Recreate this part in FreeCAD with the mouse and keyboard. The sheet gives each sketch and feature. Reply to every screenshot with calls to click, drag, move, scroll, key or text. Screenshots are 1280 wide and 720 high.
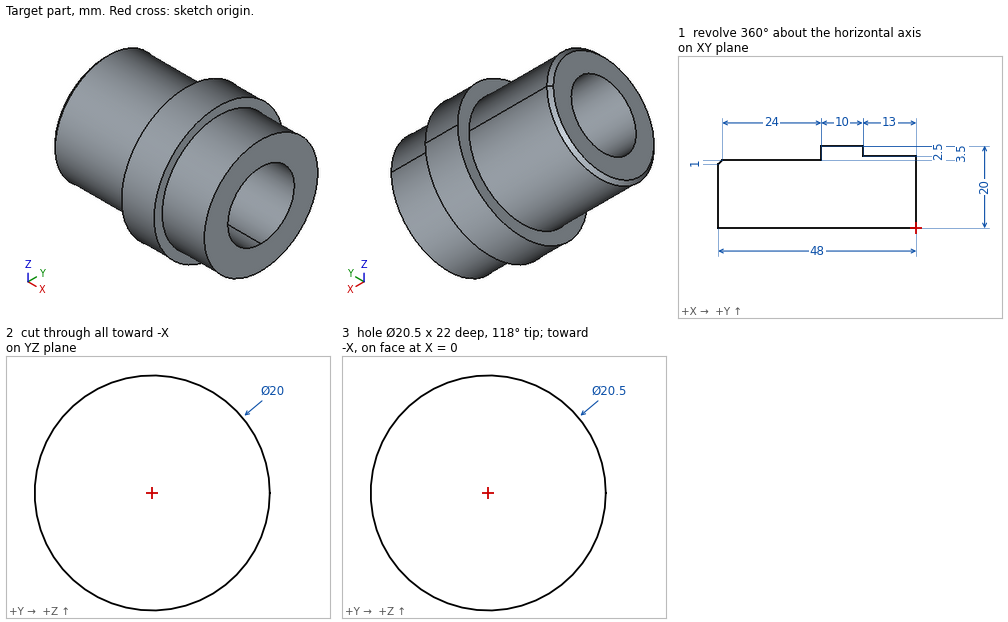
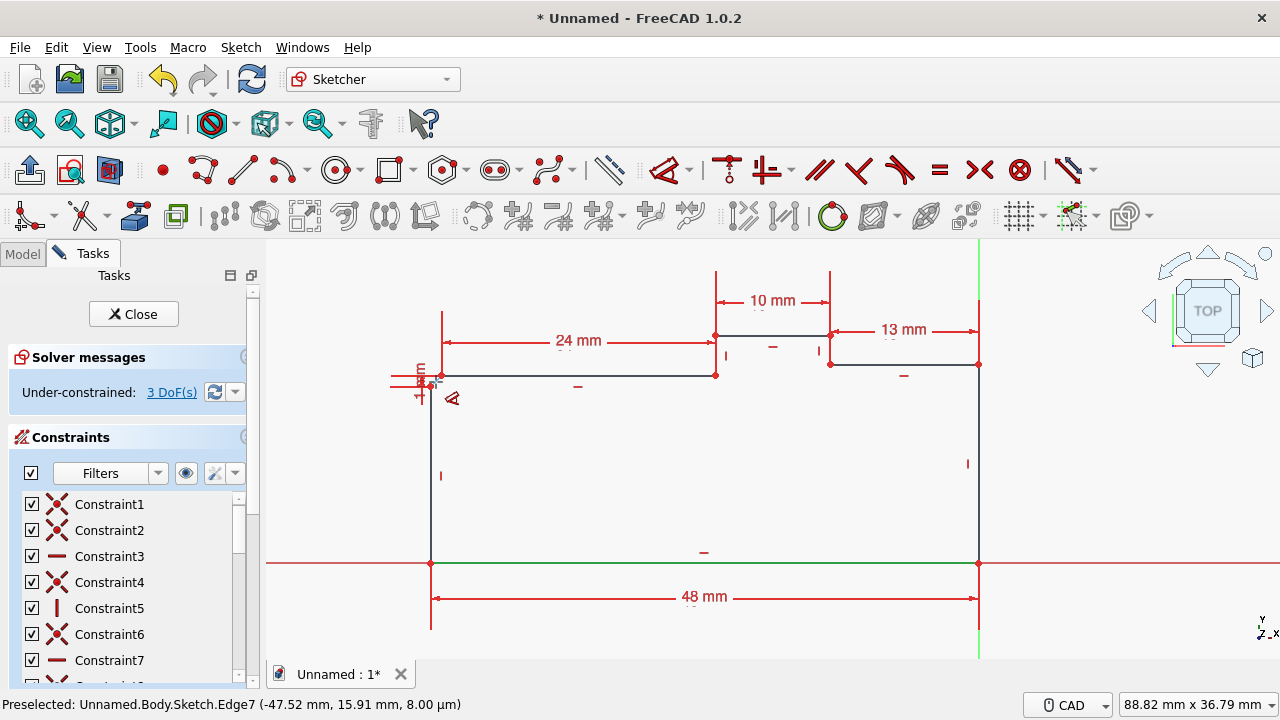
scroll(830, 356, up, 3)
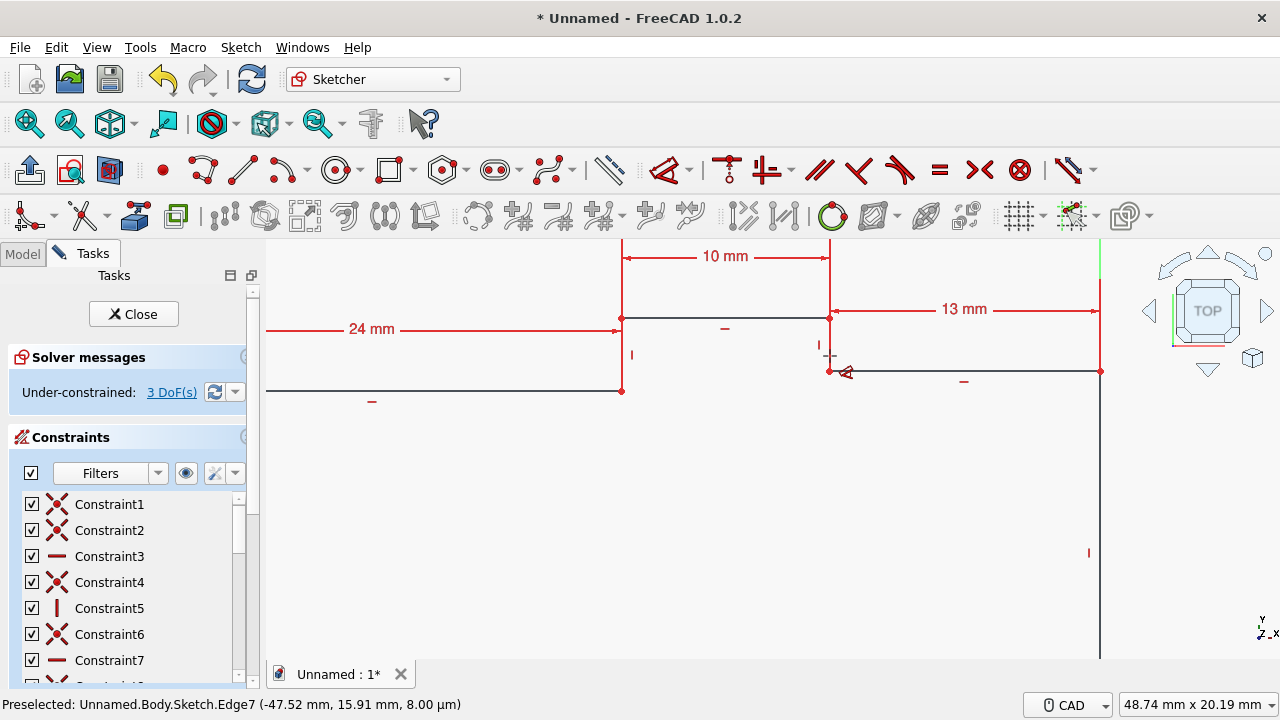
click(830, 355)
click(864, 345)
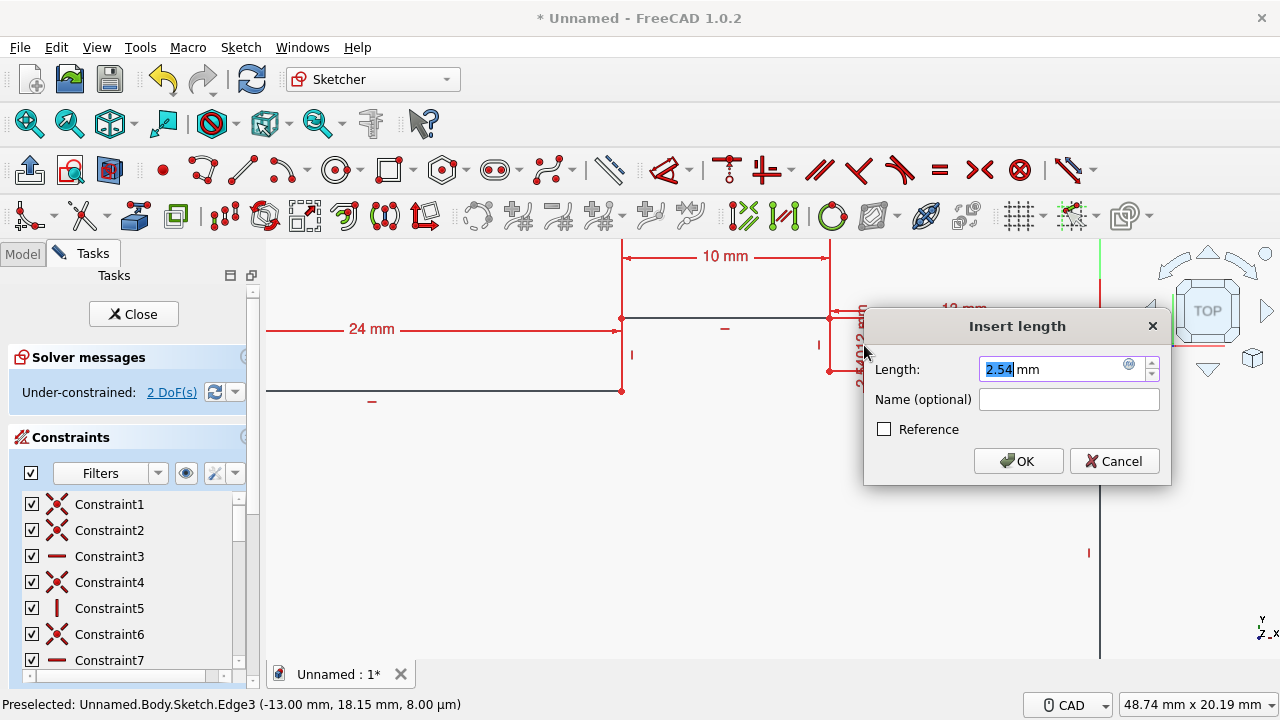
text(2.5)
key(Return)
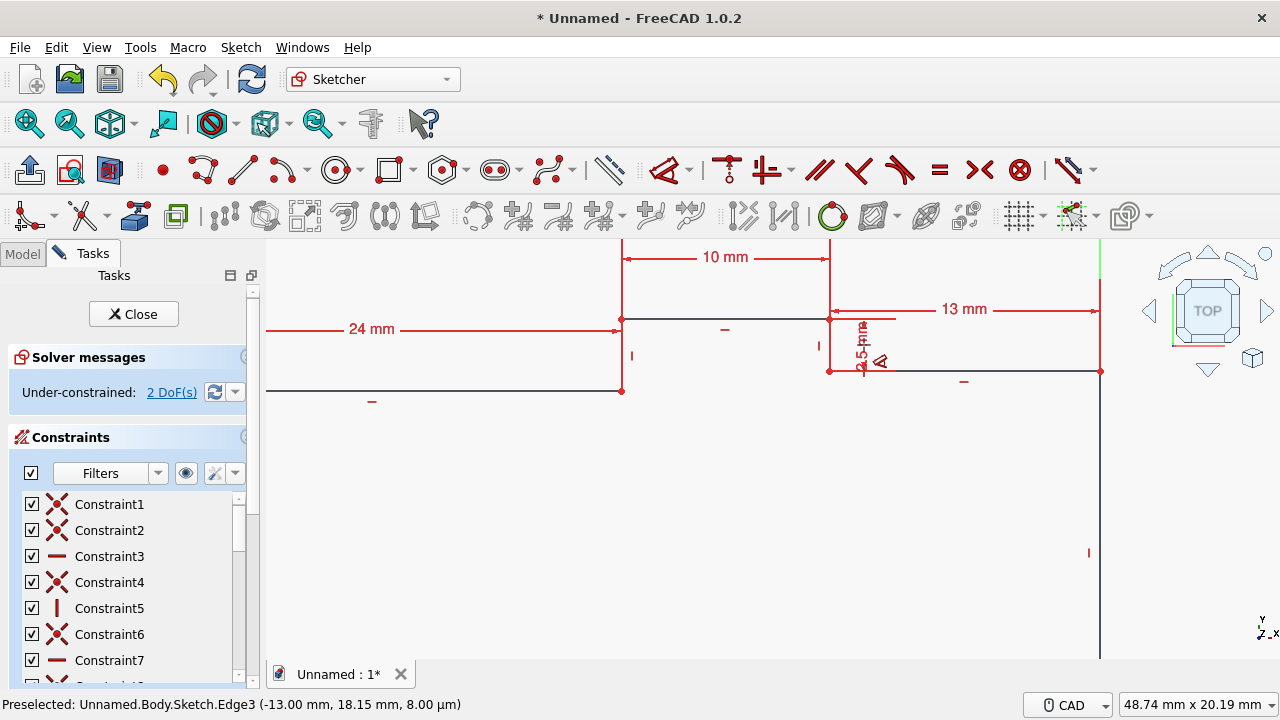
click(622, 341)
click(656, 355)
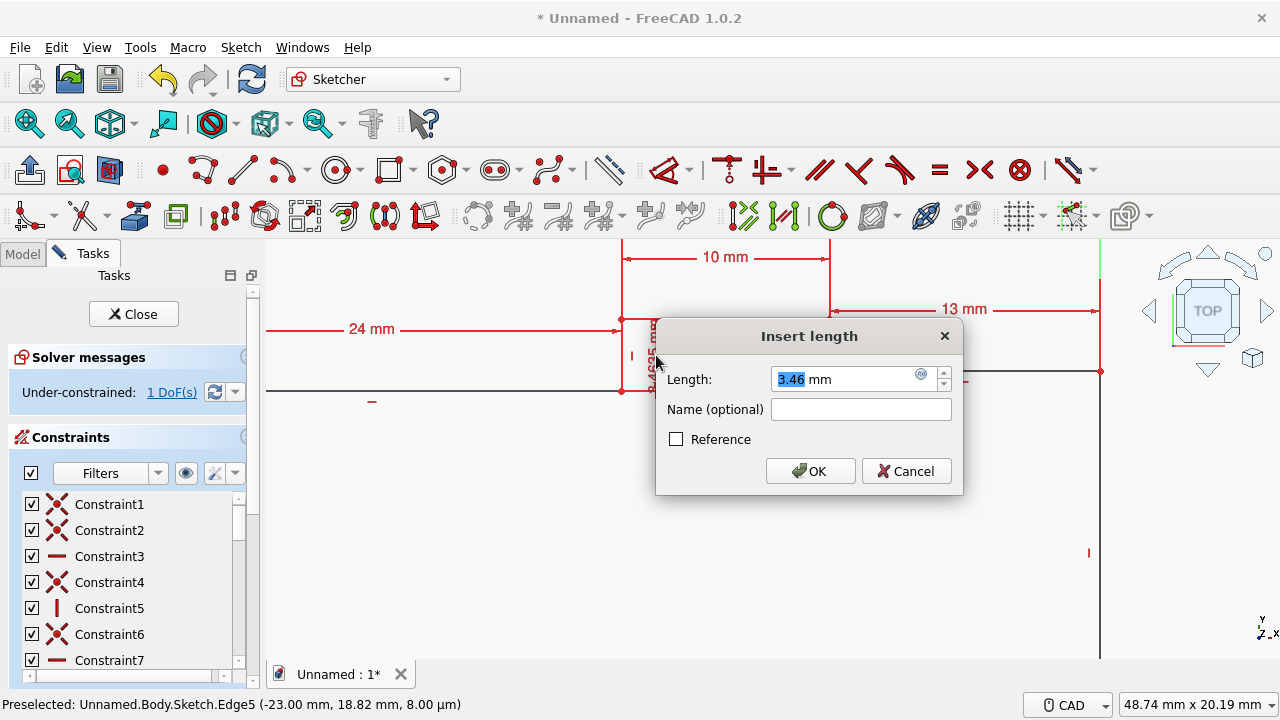
text(3.5)
key(Return)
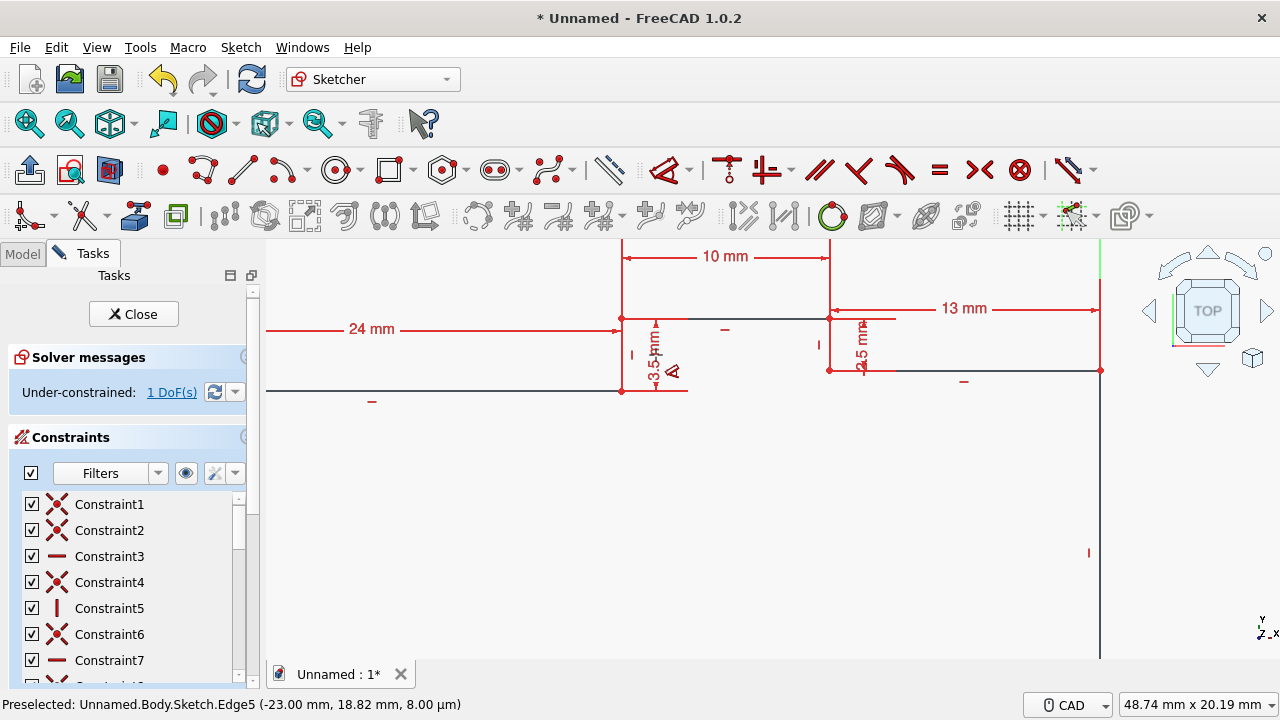
click(830, 319)
click(796, 475)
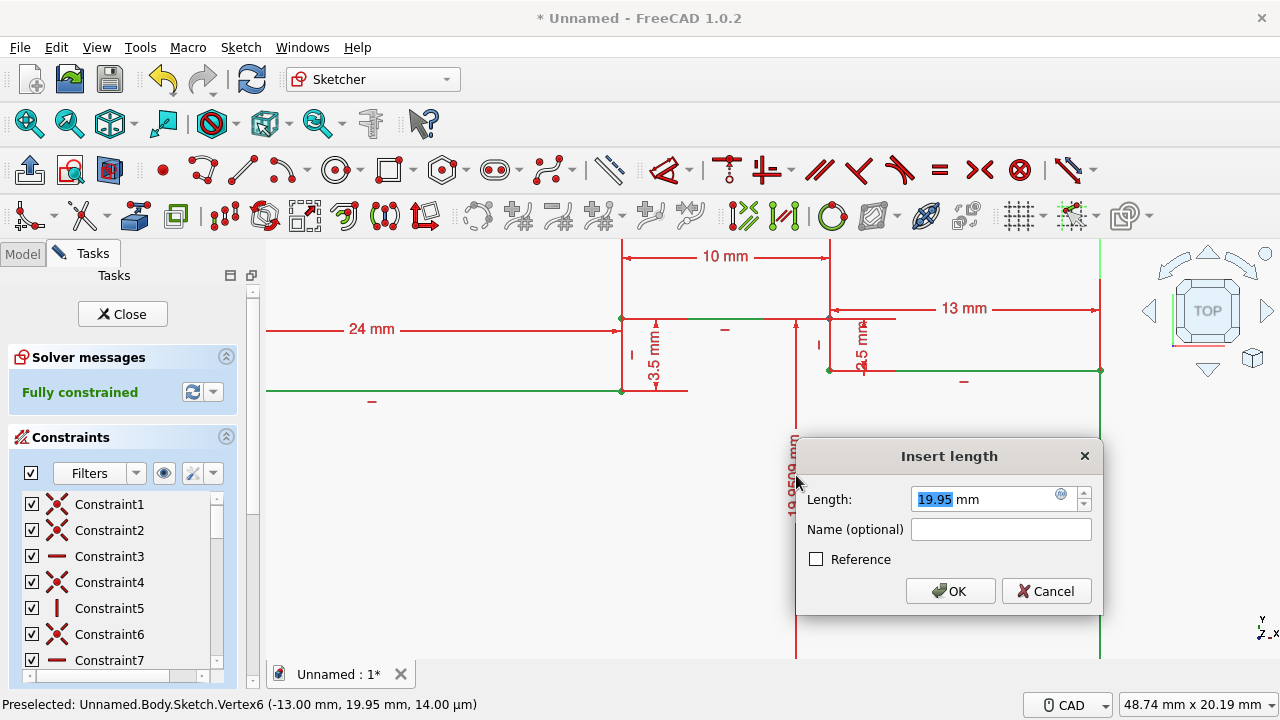
text(20)
key(Return)
key(Escape)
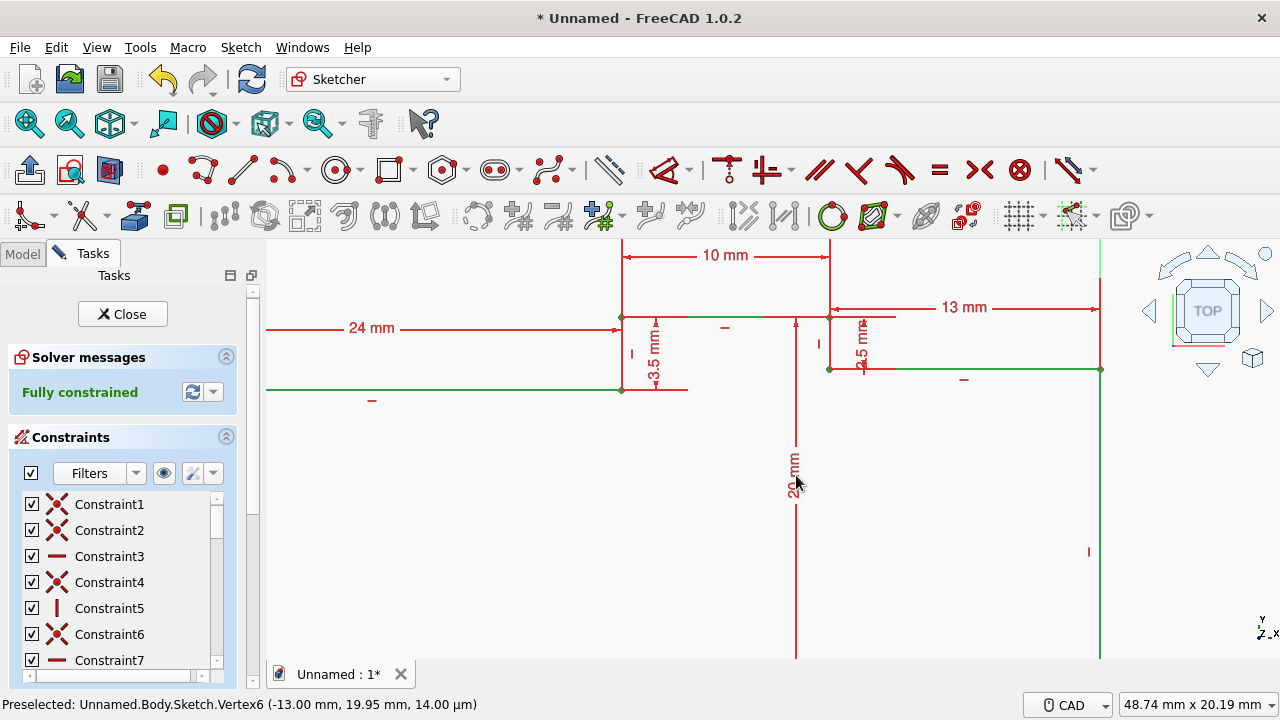
click(123, 314)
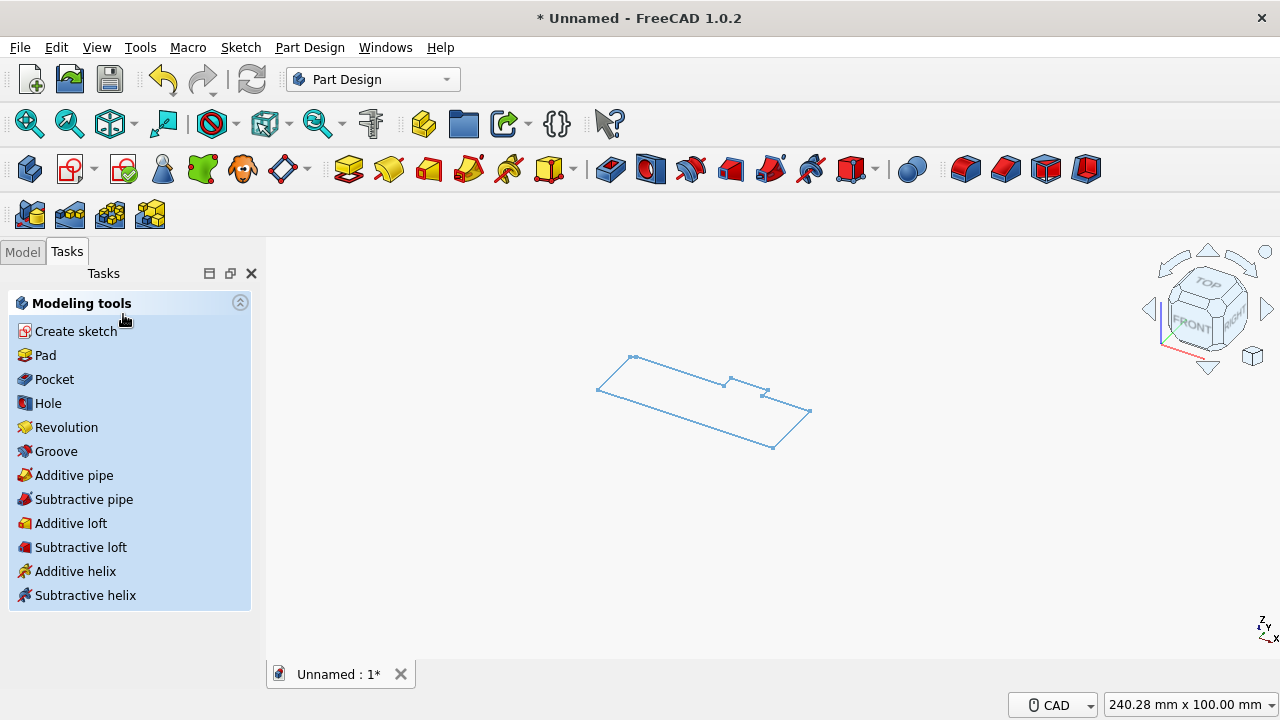
click(390, 170)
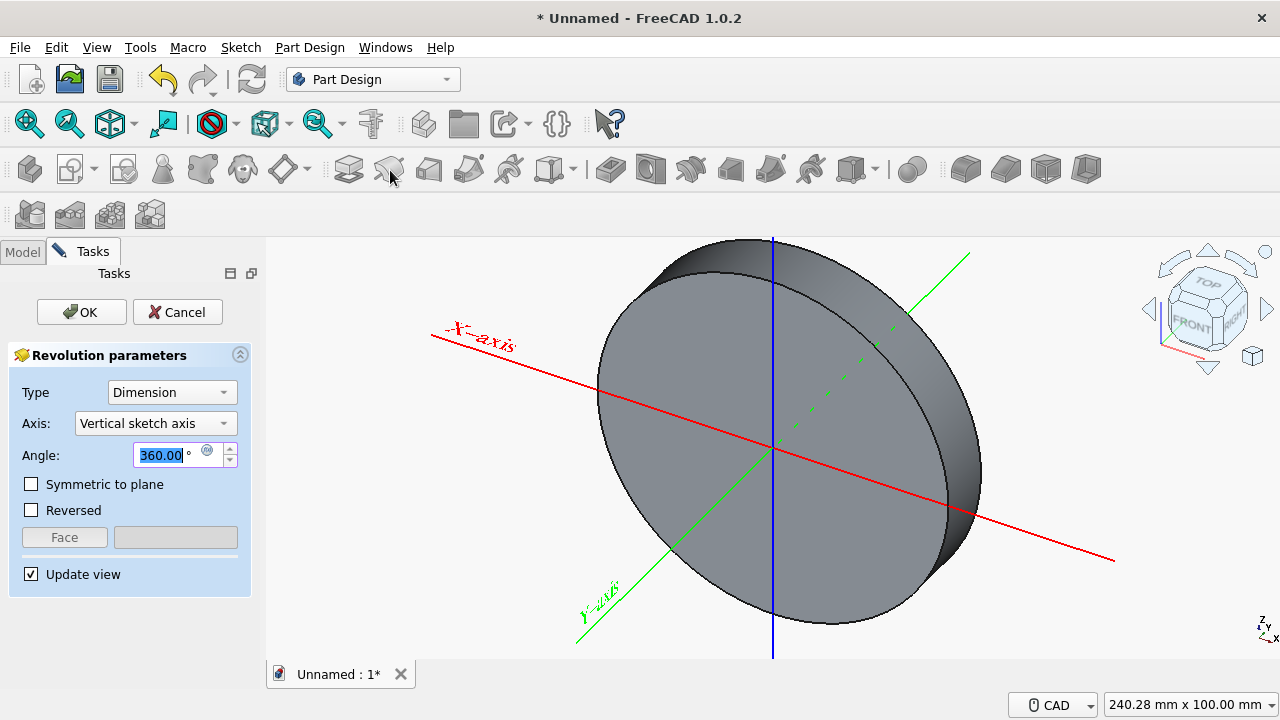
click(156, 424)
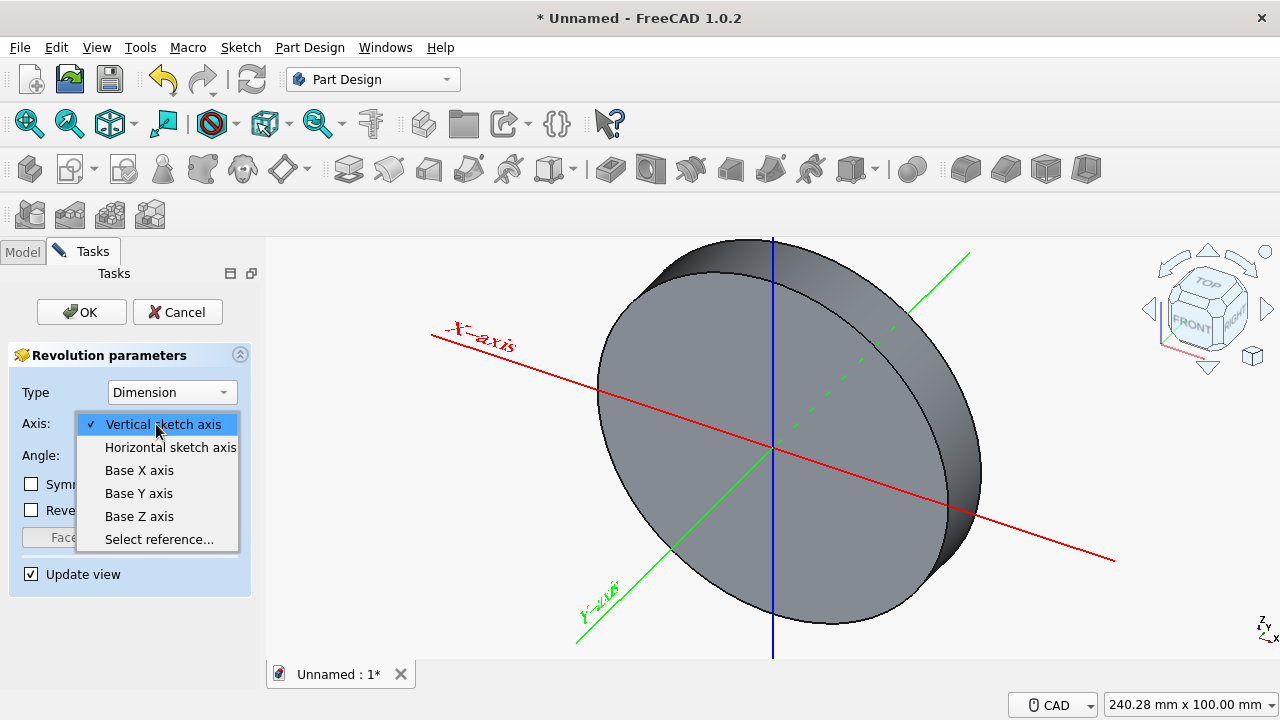
click(156, 448)